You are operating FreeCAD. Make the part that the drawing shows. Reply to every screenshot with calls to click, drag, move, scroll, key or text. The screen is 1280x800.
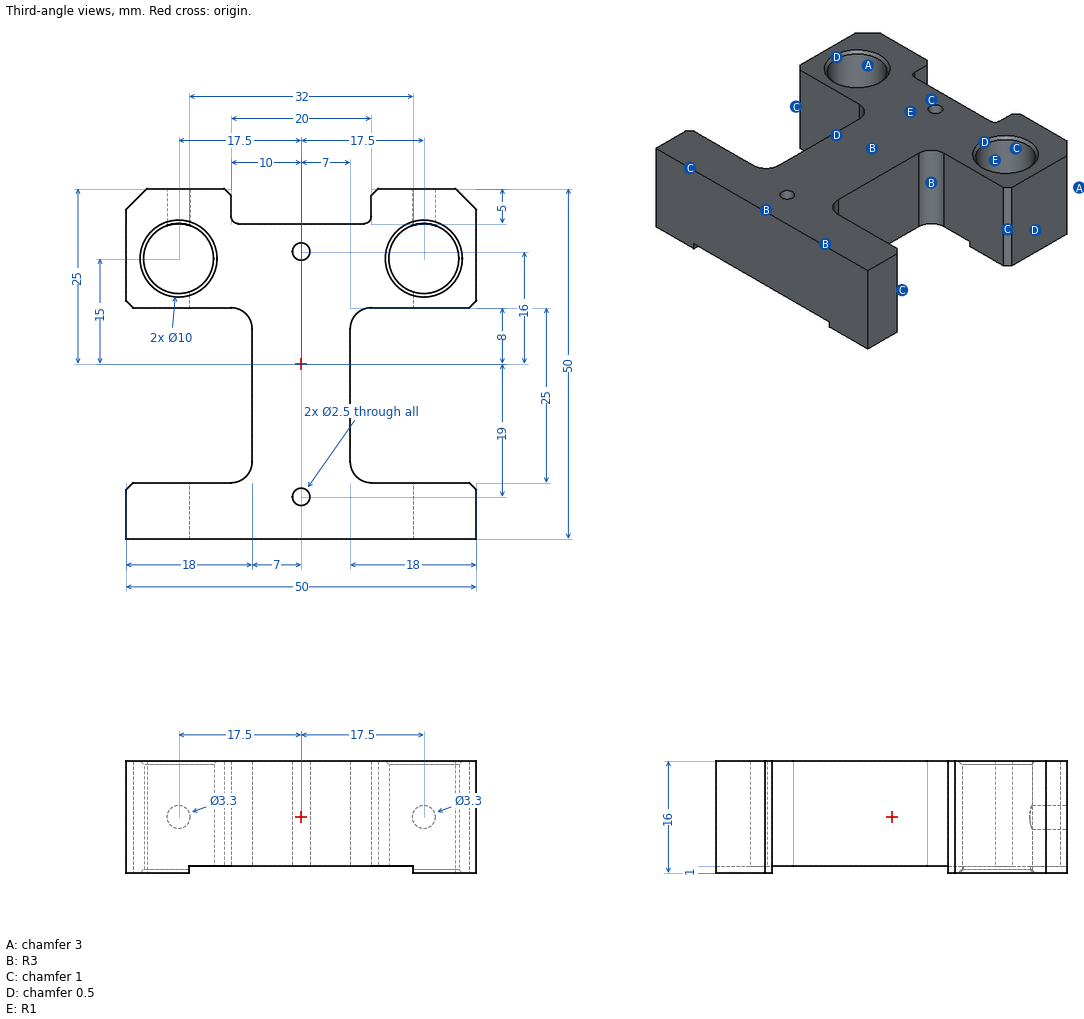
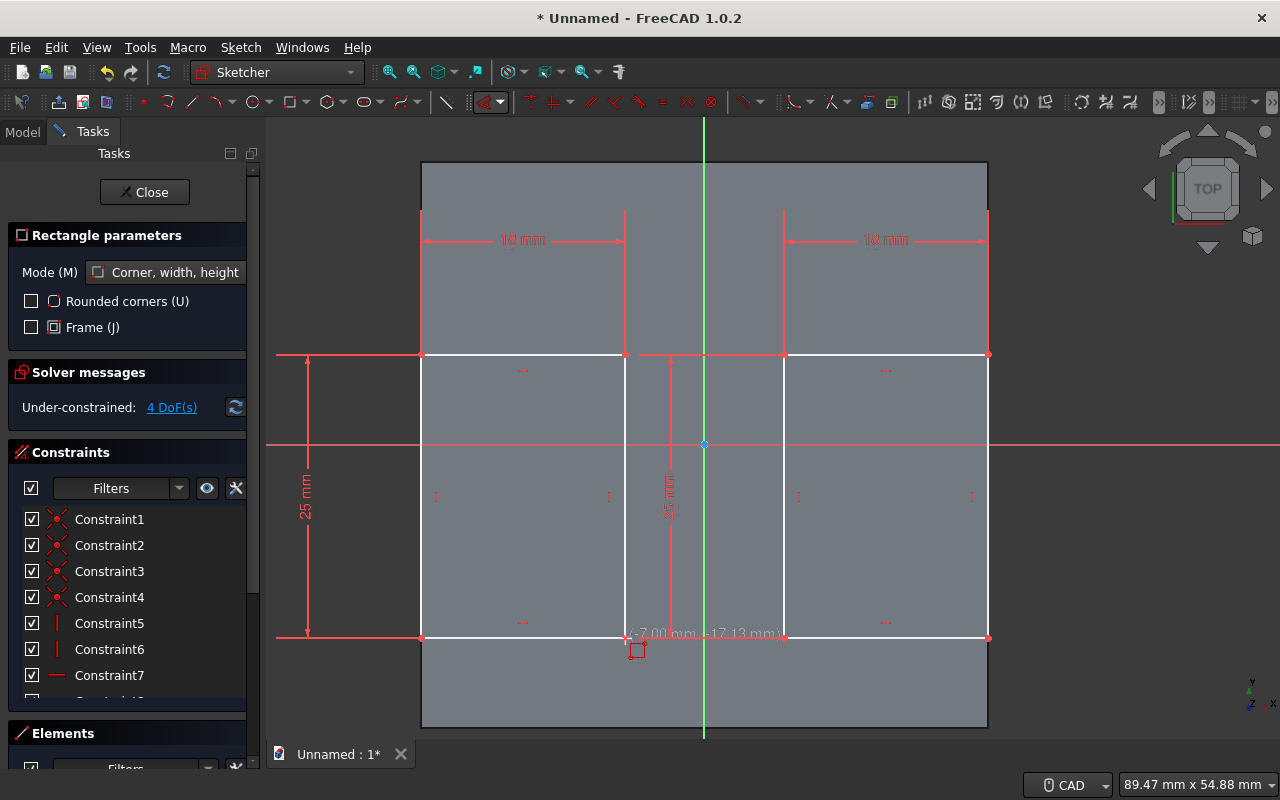
click(254, 102)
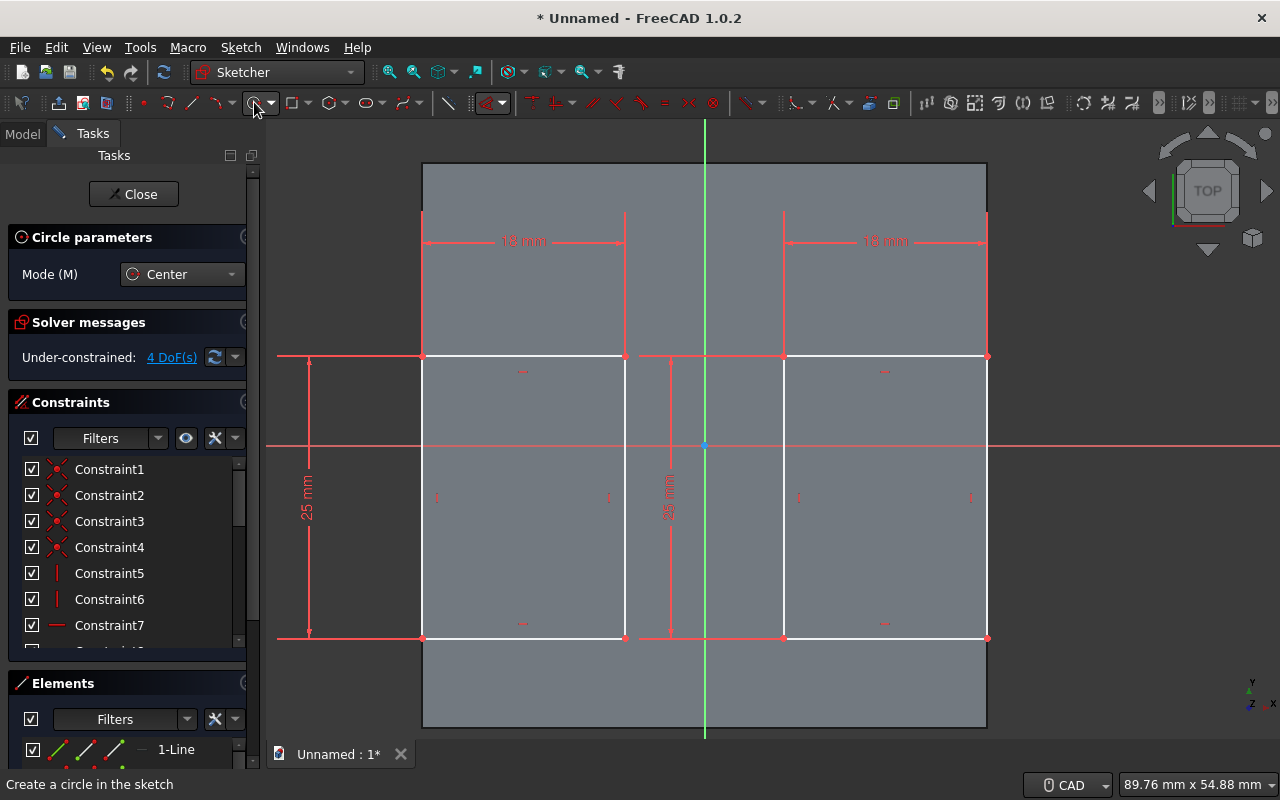
click(507, 276)
move(547, 236)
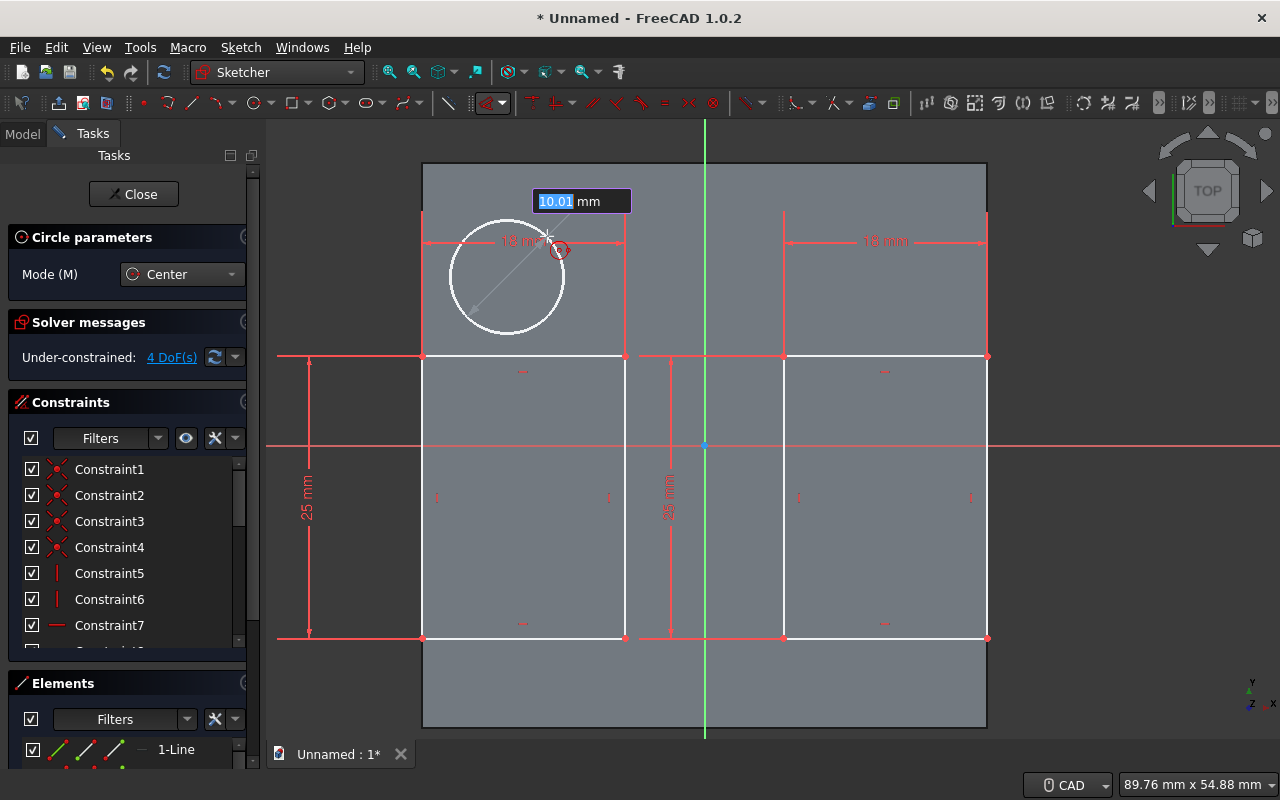
text(10)
key(Return)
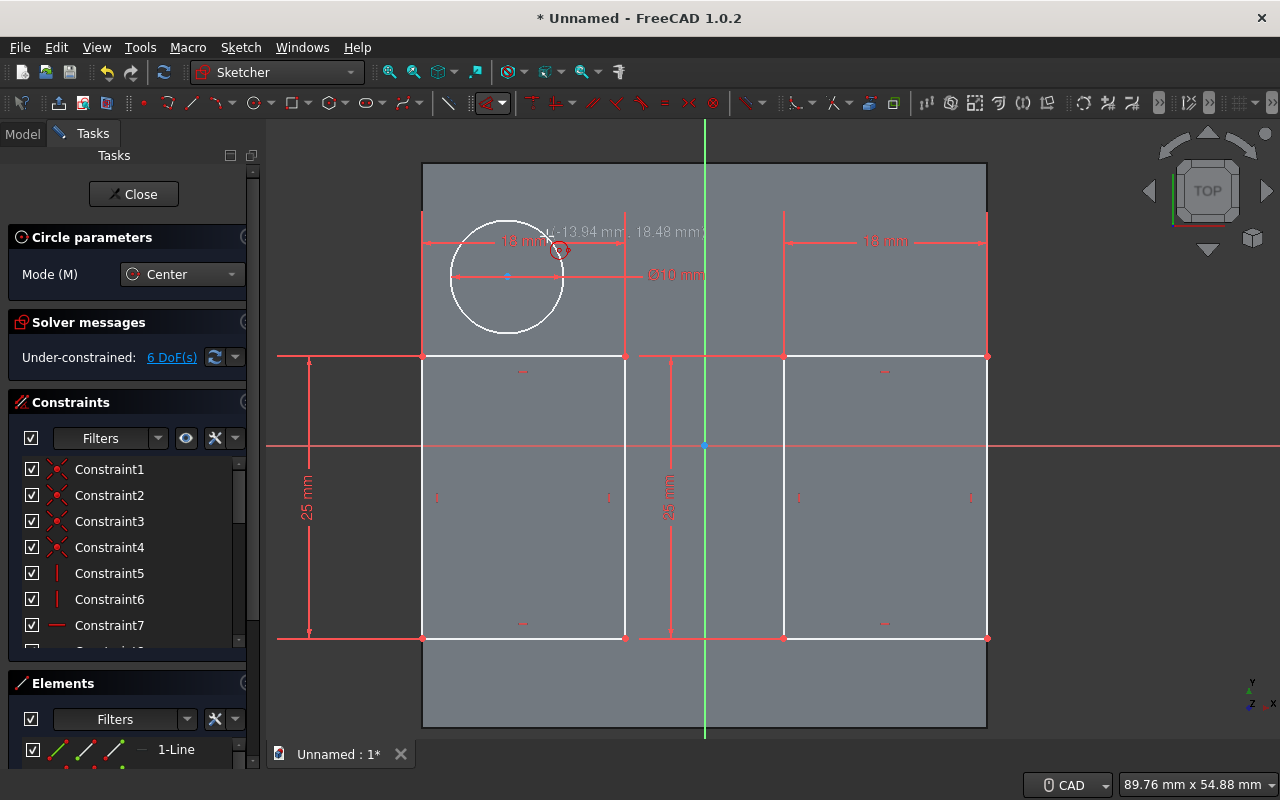
click(902, 276)
move(942, 236)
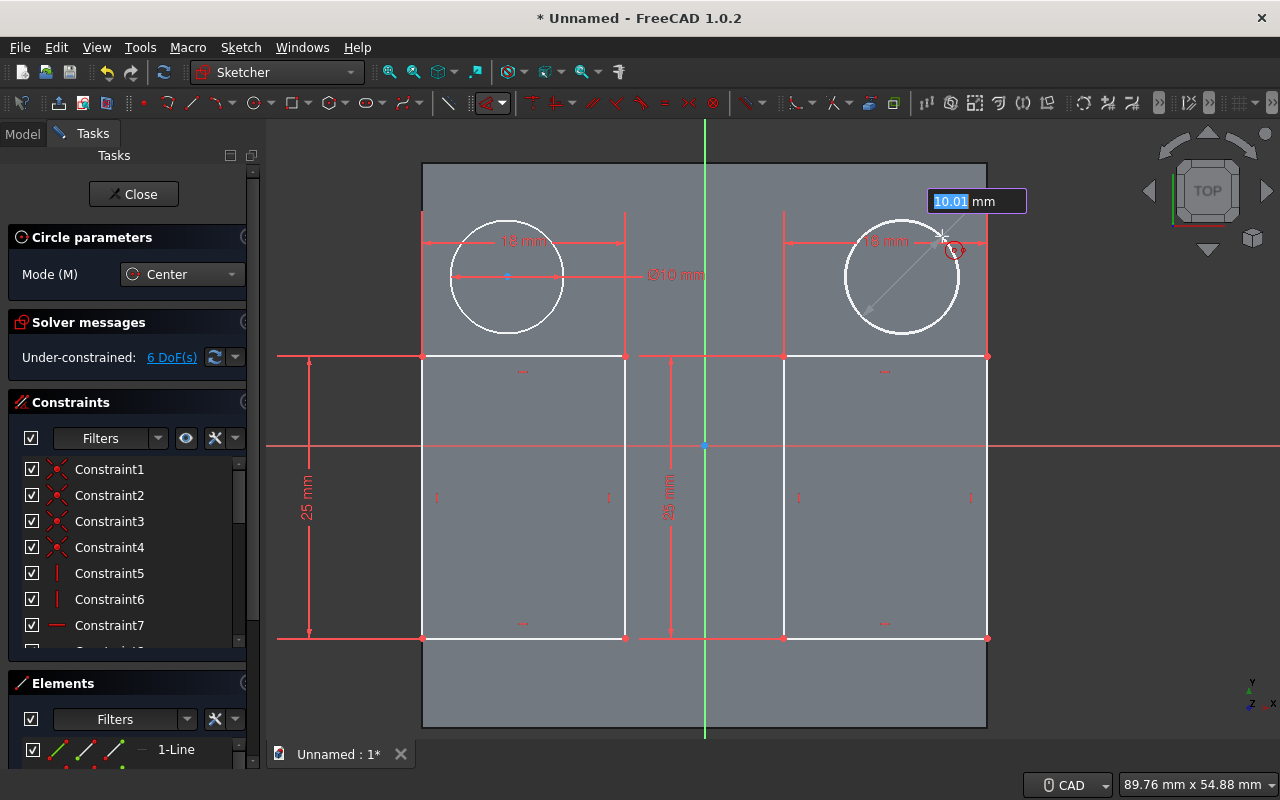
text(10)
key(Return)
key(Escape)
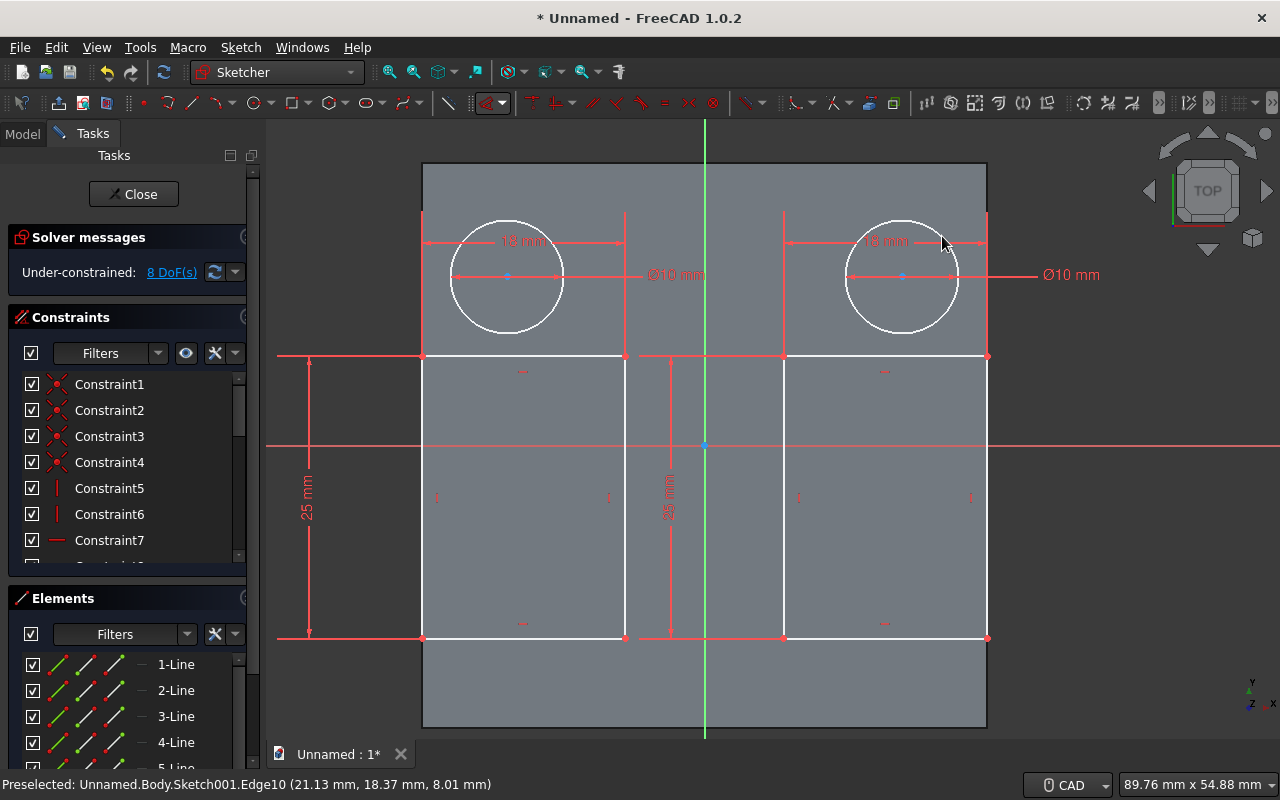
key(d)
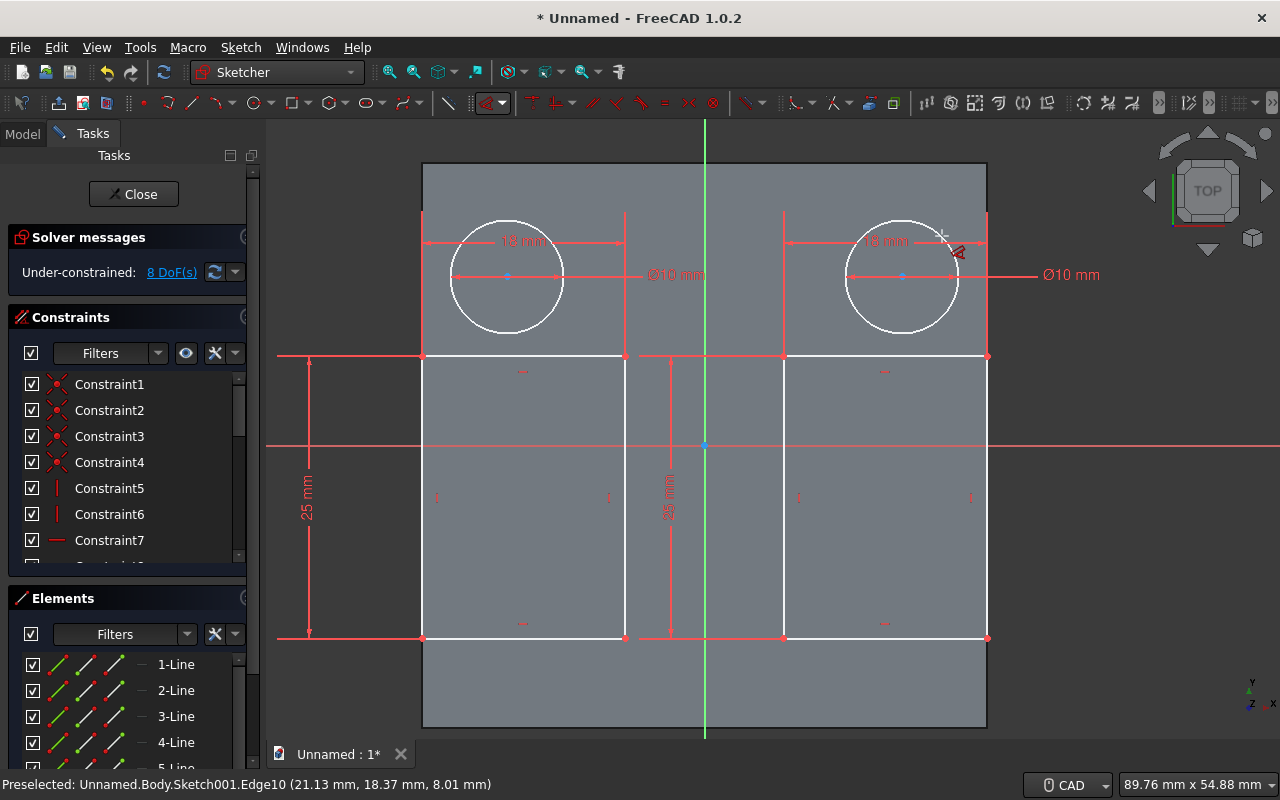
click(784, 356)
click(744, 322)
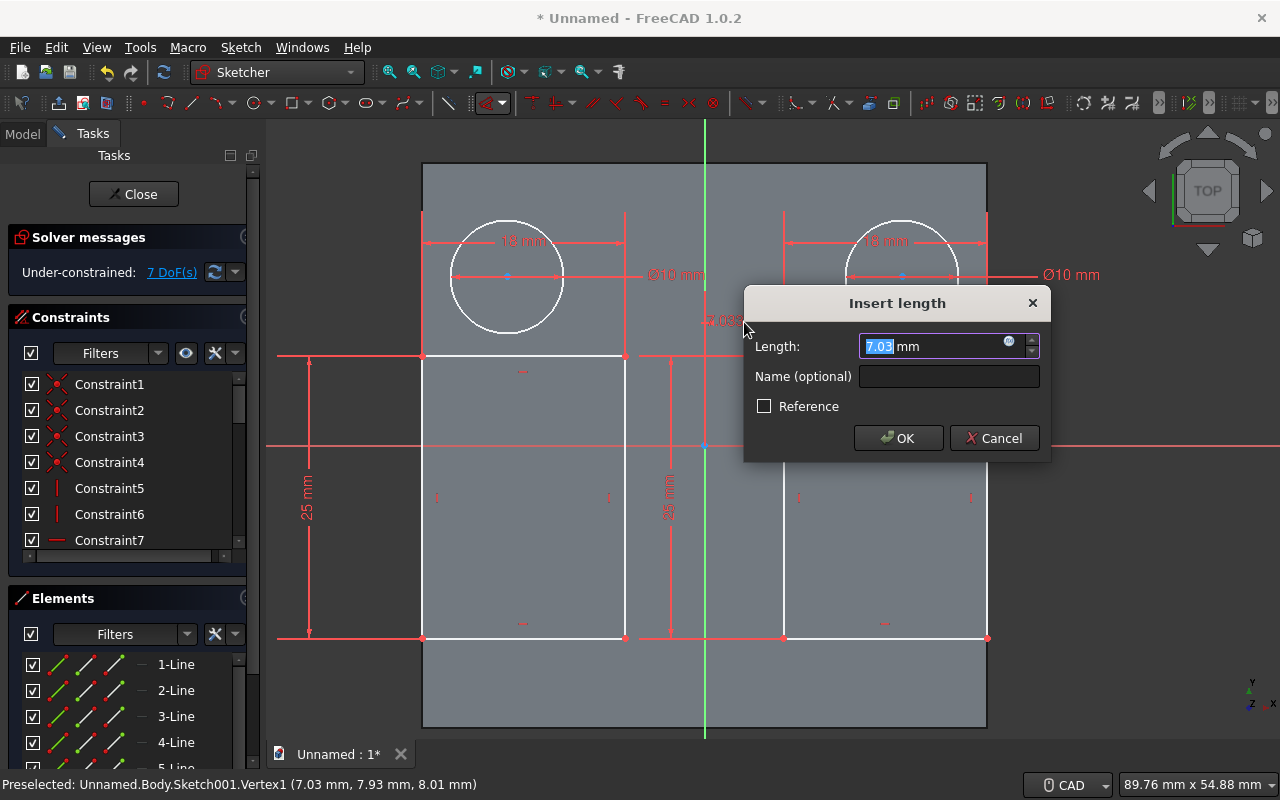
text(7)
key(Return)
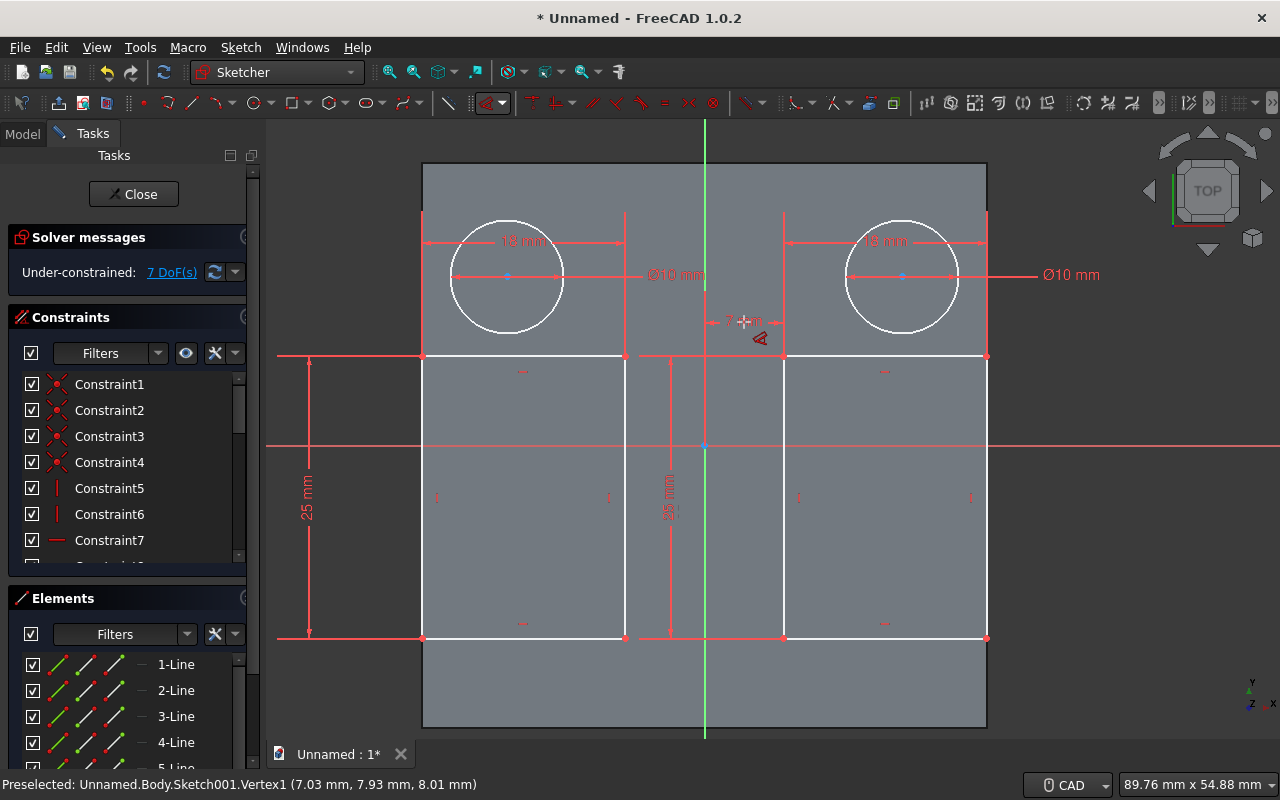
click(784, 356)
click(818, 401)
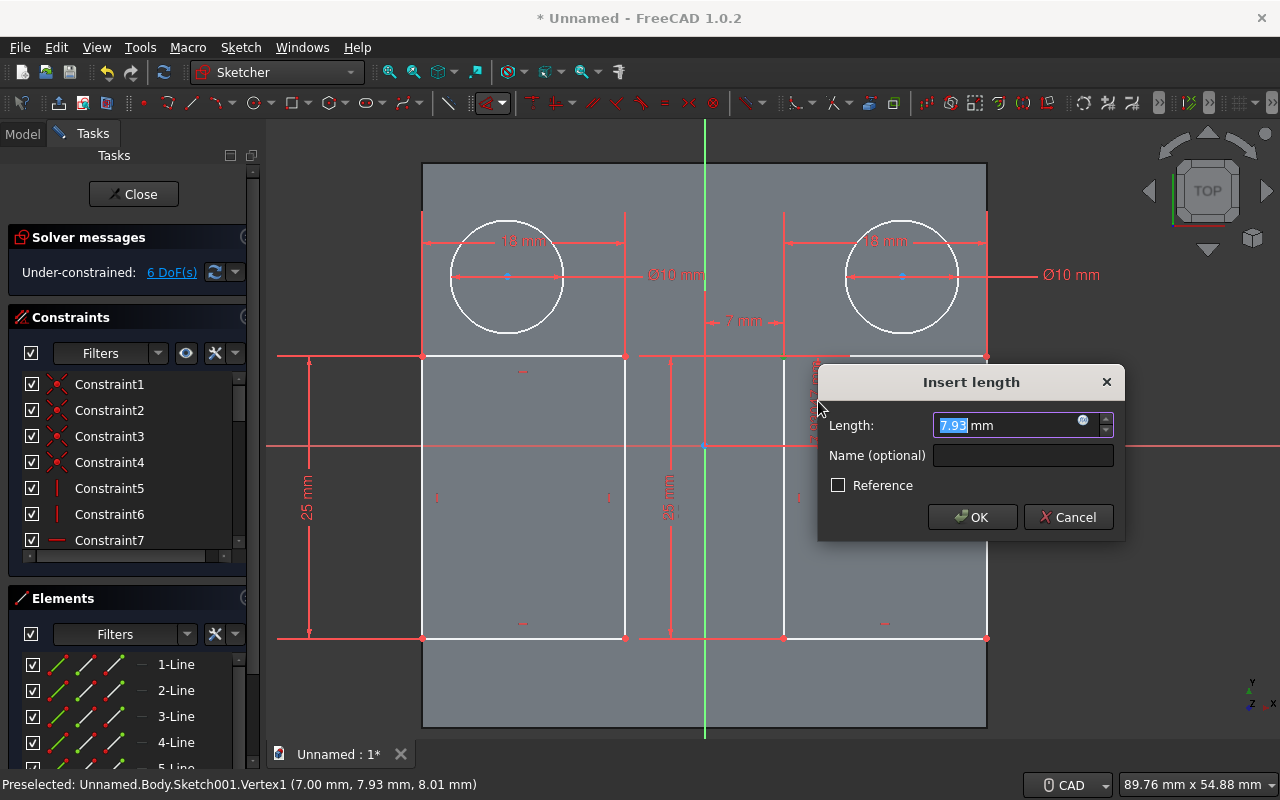
text(8)
key(Return)